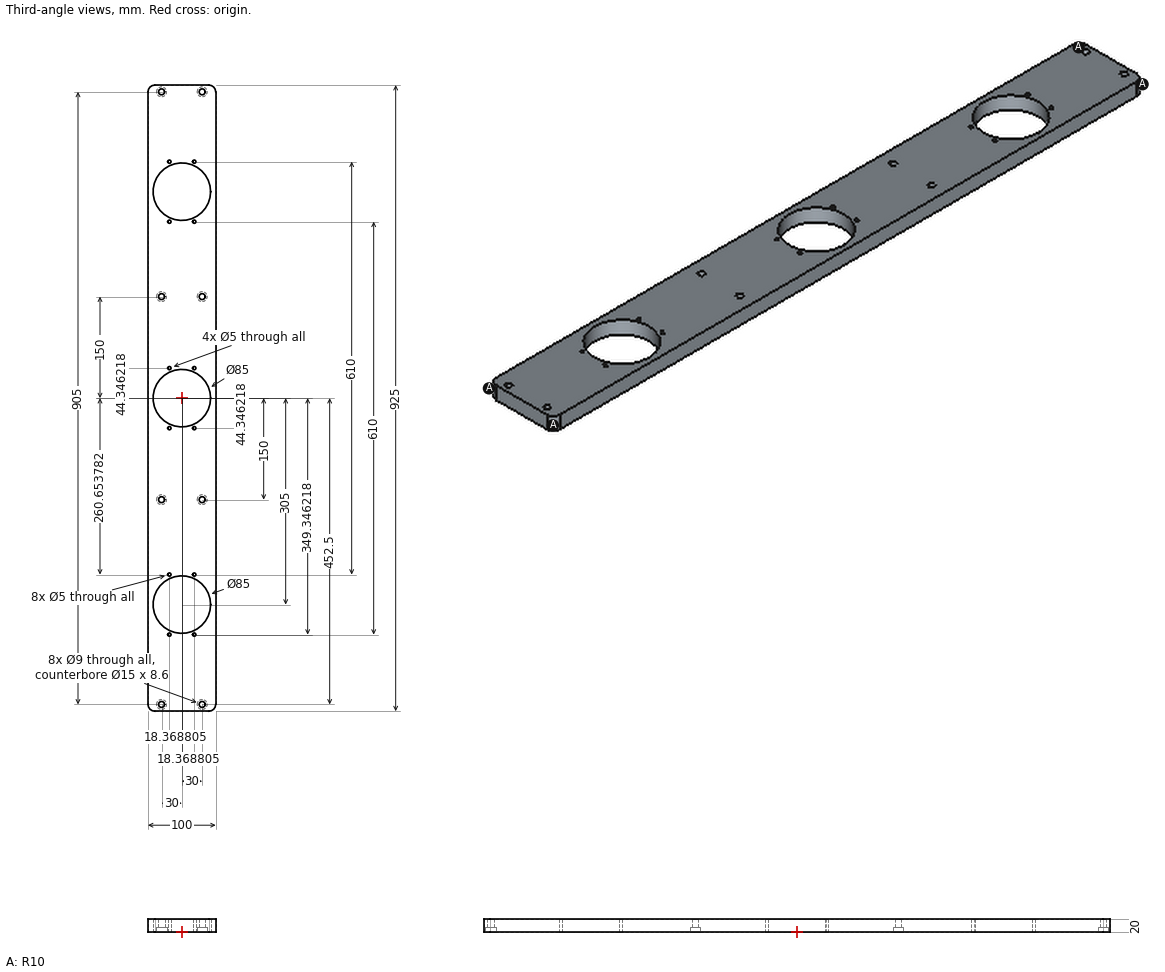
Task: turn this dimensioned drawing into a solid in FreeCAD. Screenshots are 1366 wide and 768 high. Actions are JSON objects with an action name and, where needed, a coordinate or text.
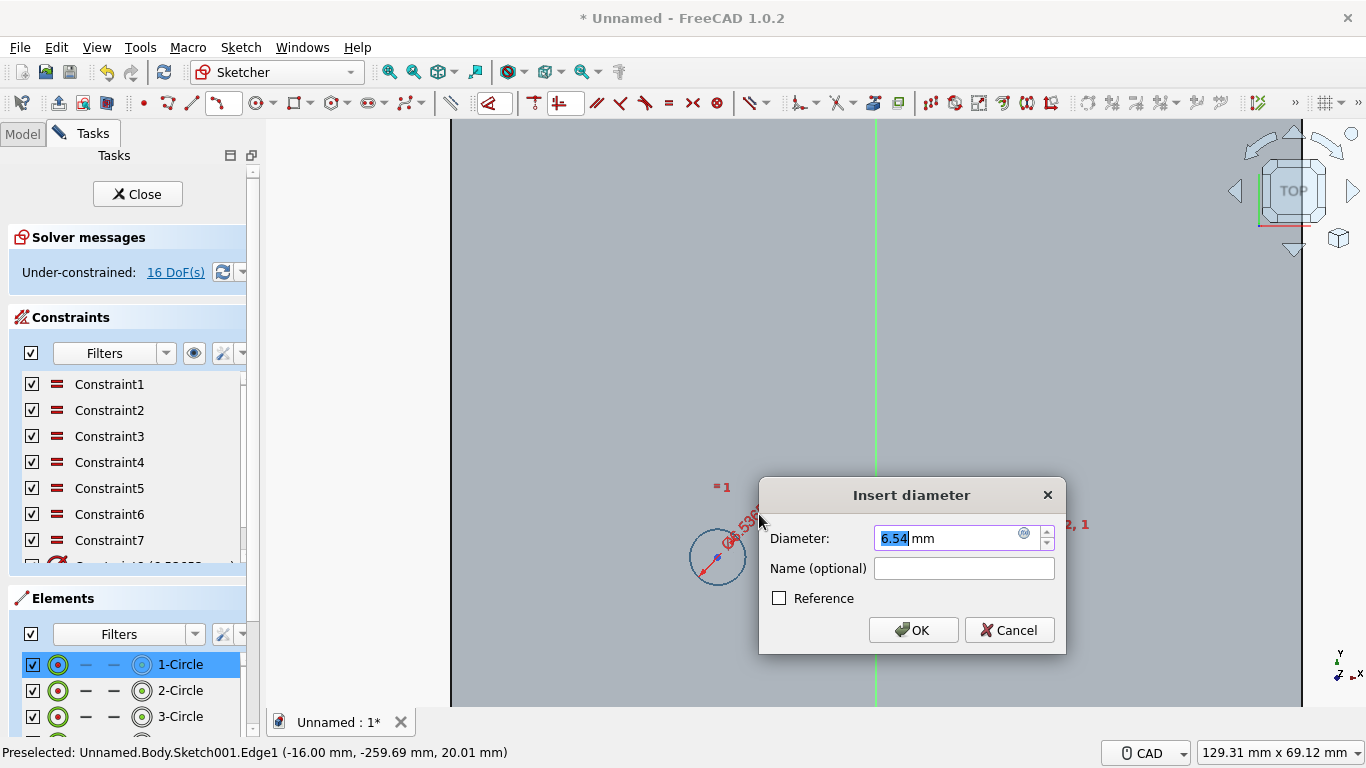
{"action": "type", "text": "5"}
{"action": "key", "text": "Return"}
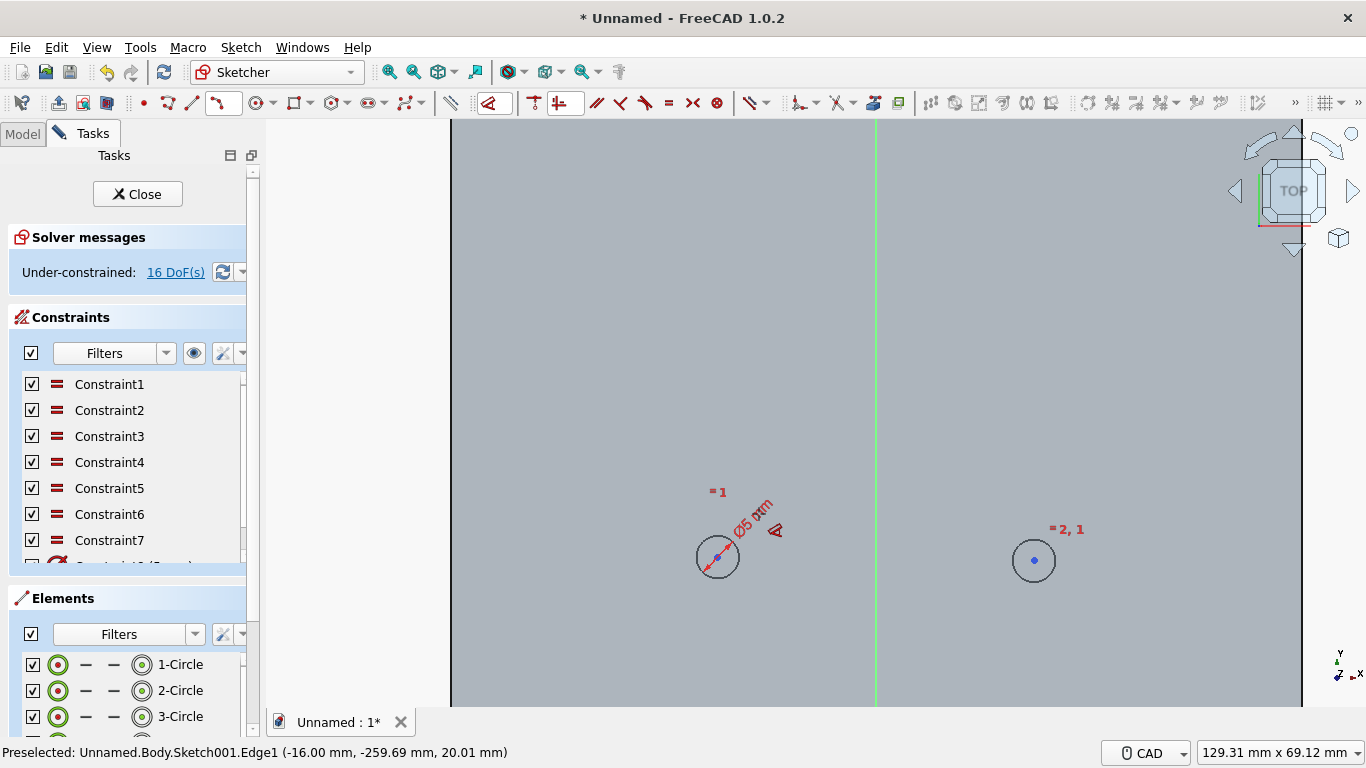
{"action": "scroll", "coordinate": [739, 548], "scroll_direction": "down", "scroll_amount": 14}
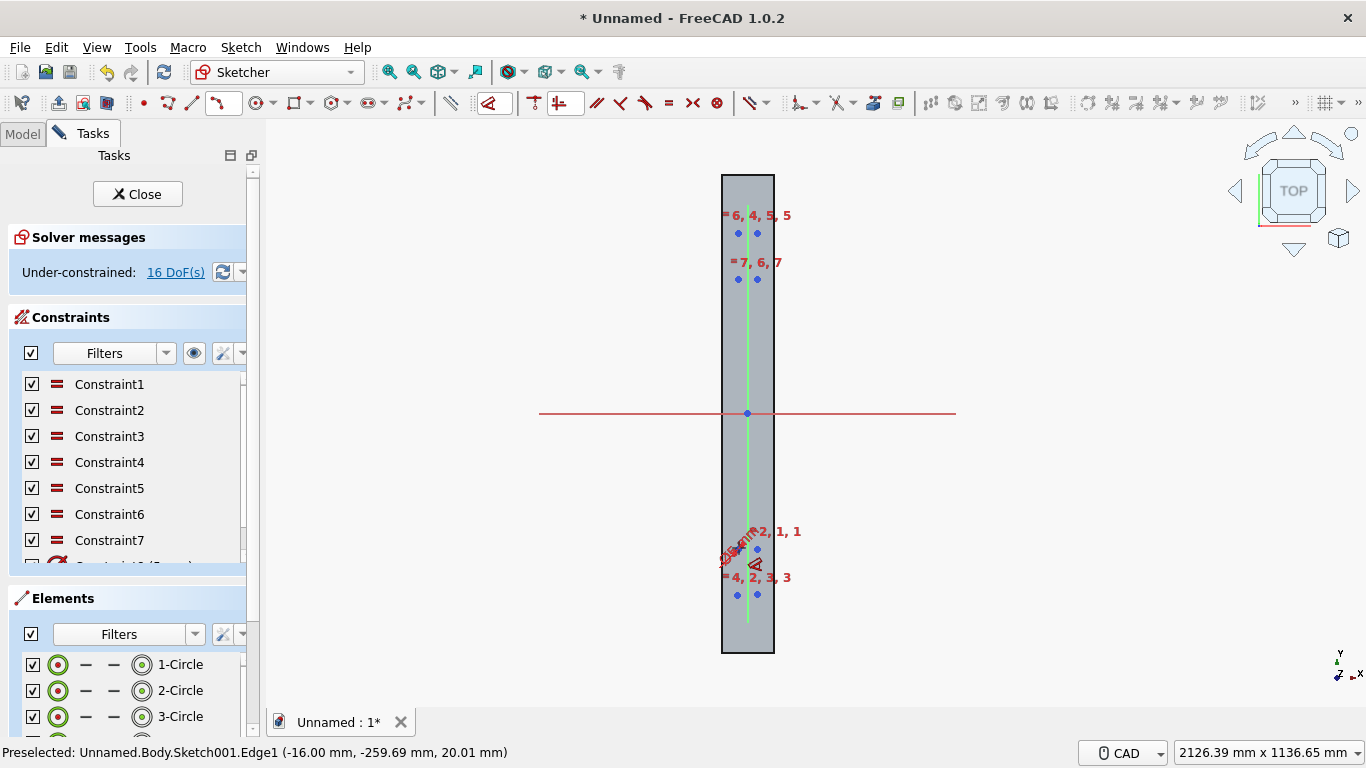
{"action": "left_click", "coordinate": [757, 549]}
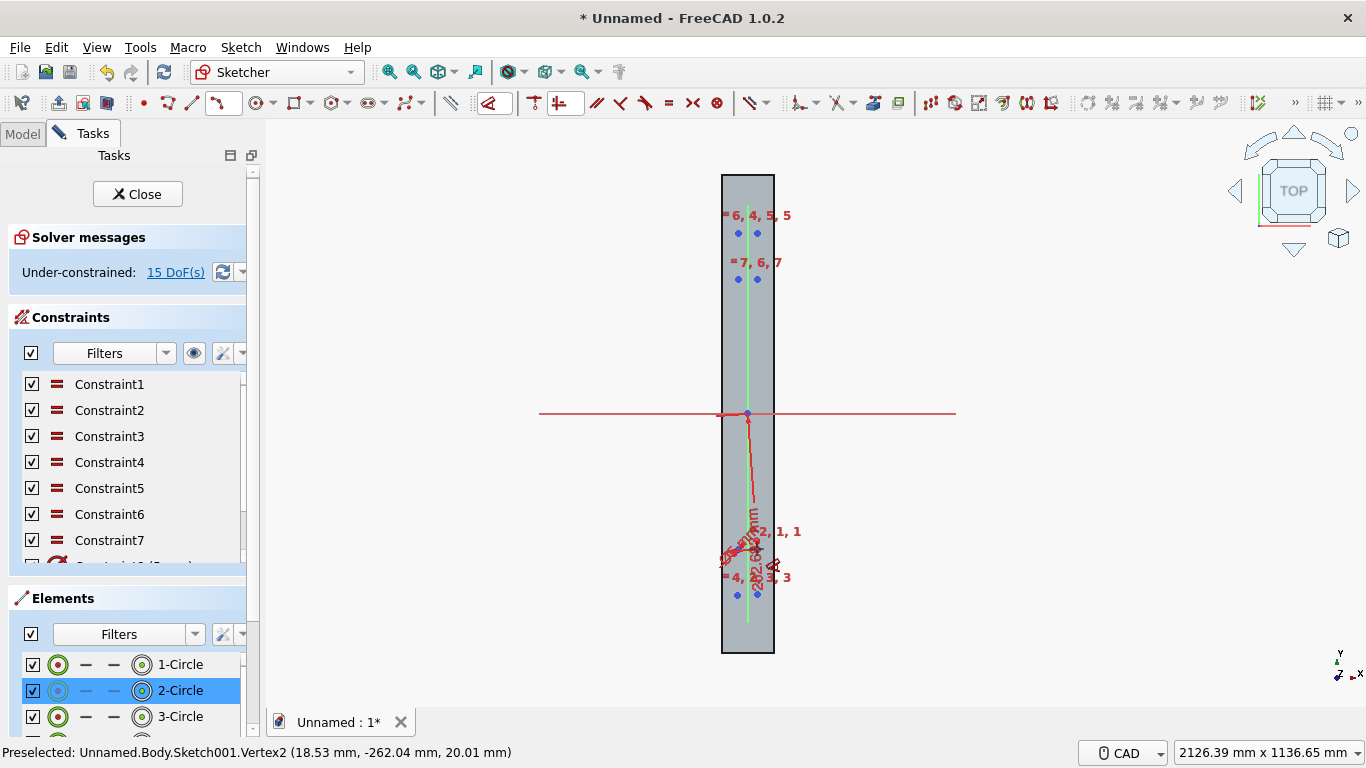
{"action": "left_click", "coordinate": [757, 234]}
{"action": "left_click", "coordinate": [791, 392]}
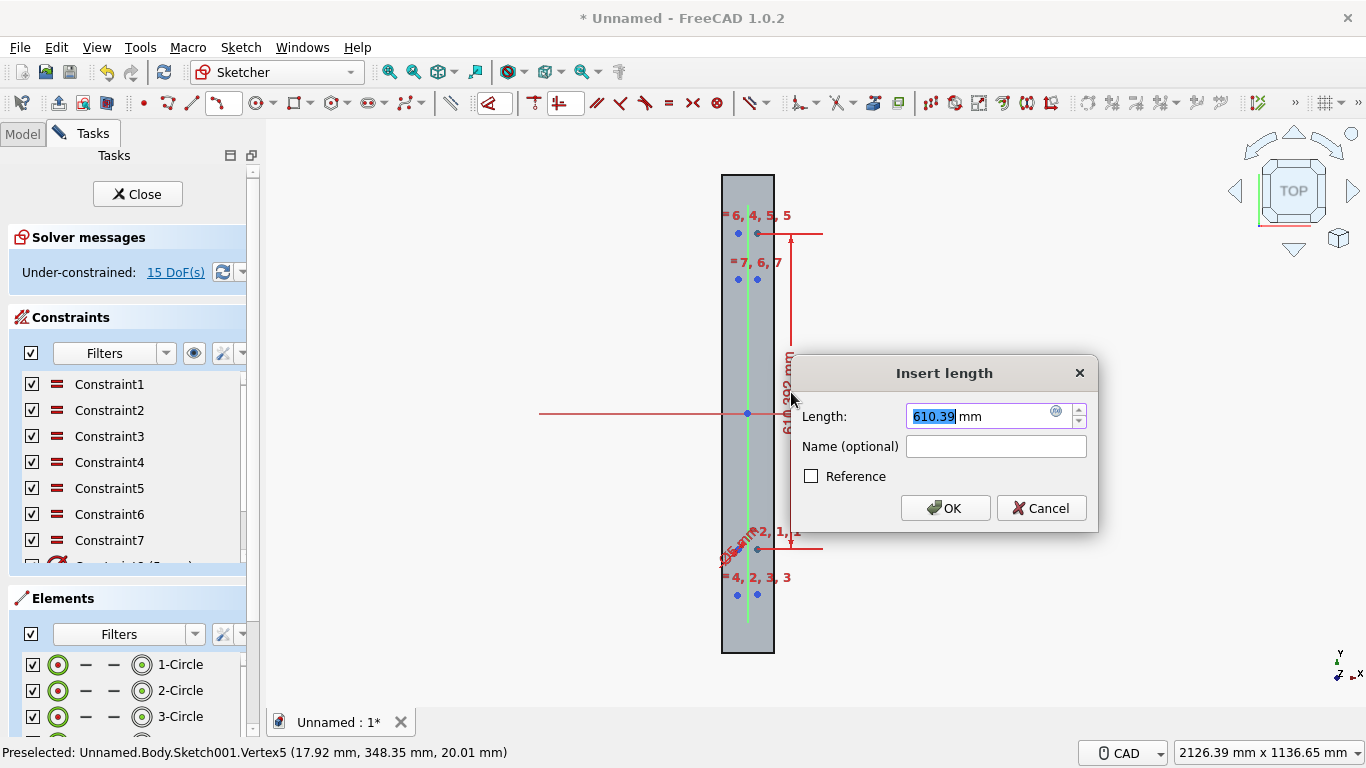
{"action": "type", "text": "610"}
{"action": "key", "text": "Return"}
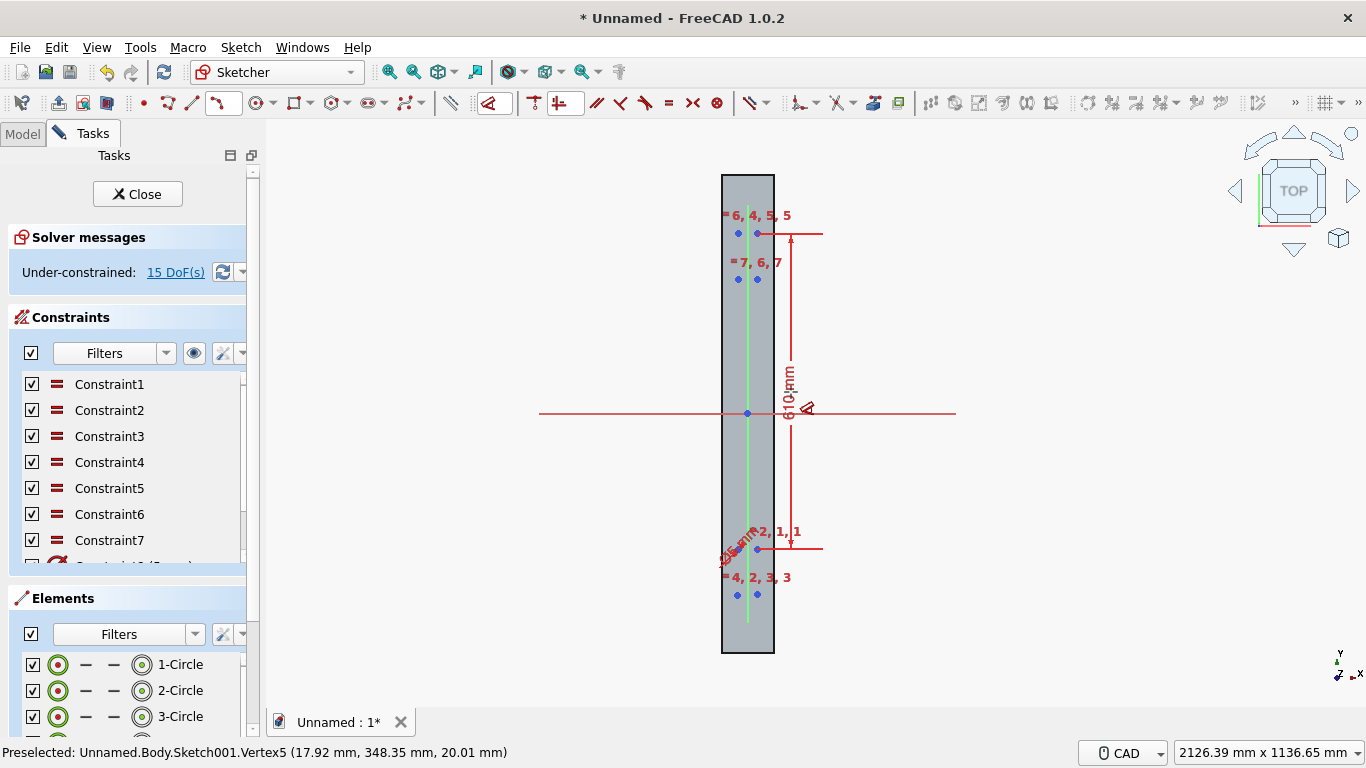
{"action": "left_click", "coordinate": [738, 549]}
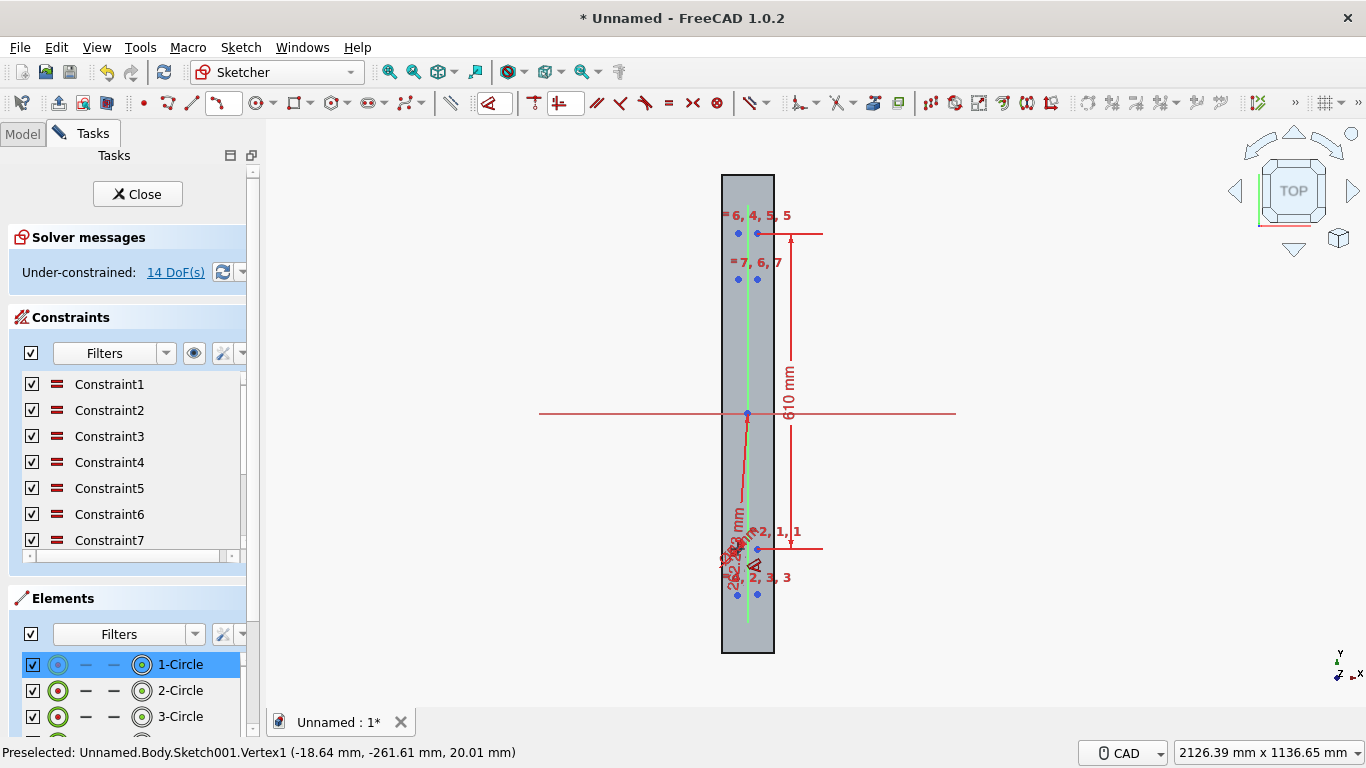
{"action": "left_click", "coordinate": [757, 234]}
{"action": "left_click", "coordinate": [704, 391]}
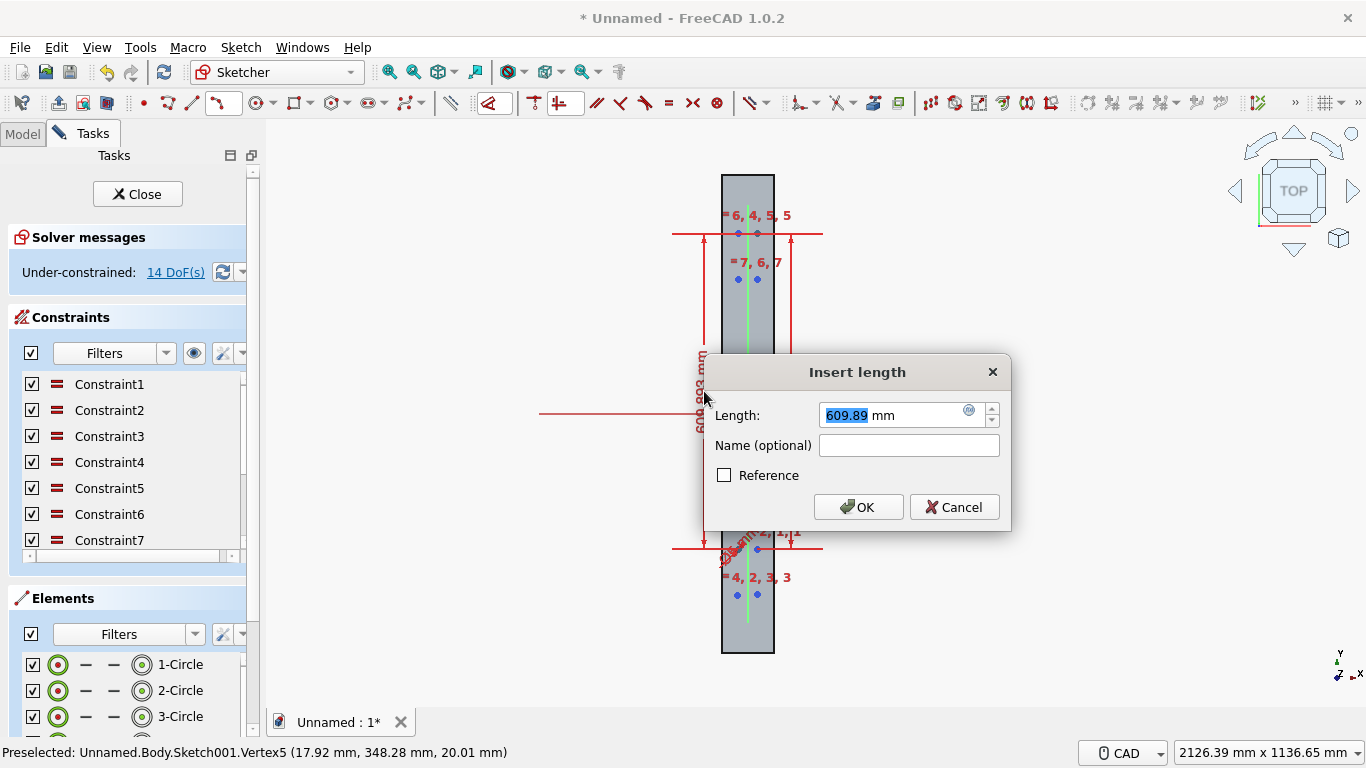
{"action": "type", "text": "610"}
{"action": "key", "text": "Return"}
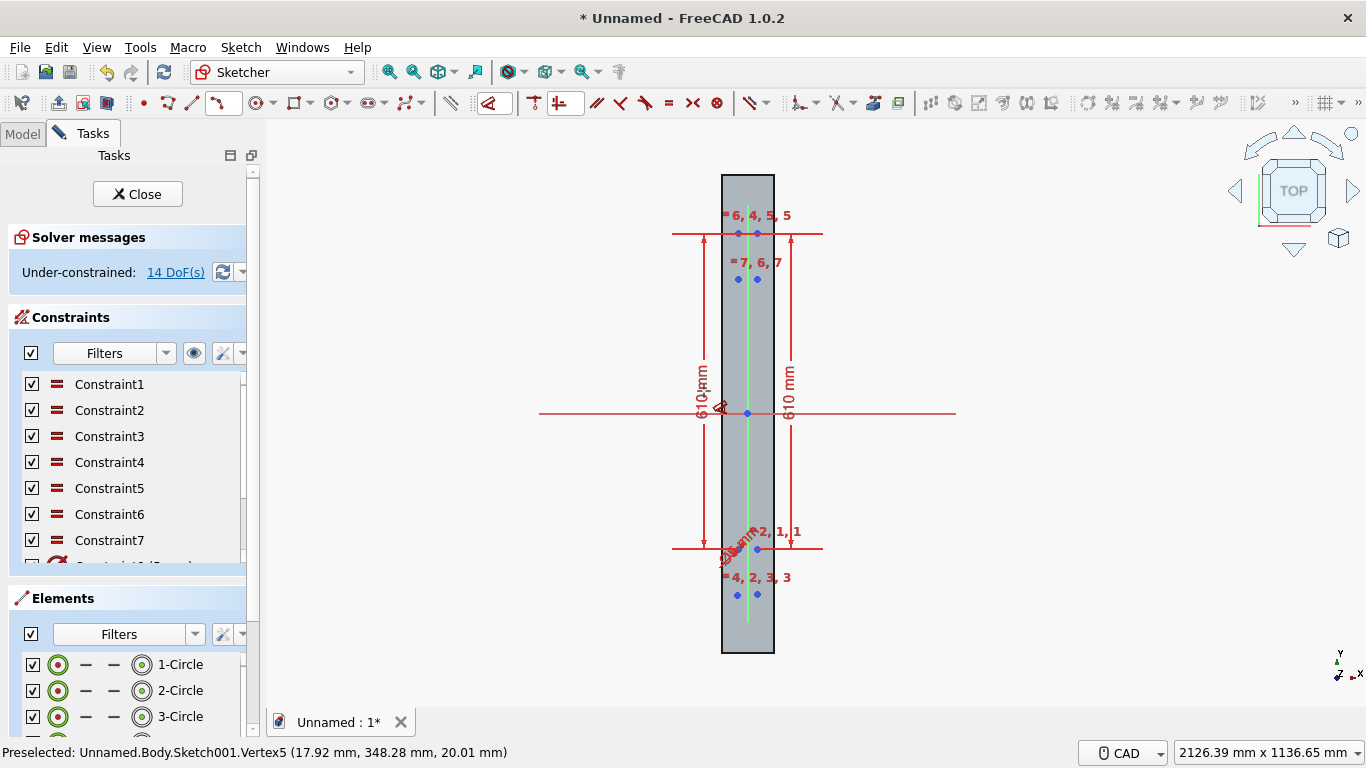
{"action": "left_click", "coordinate": [738, 549]}